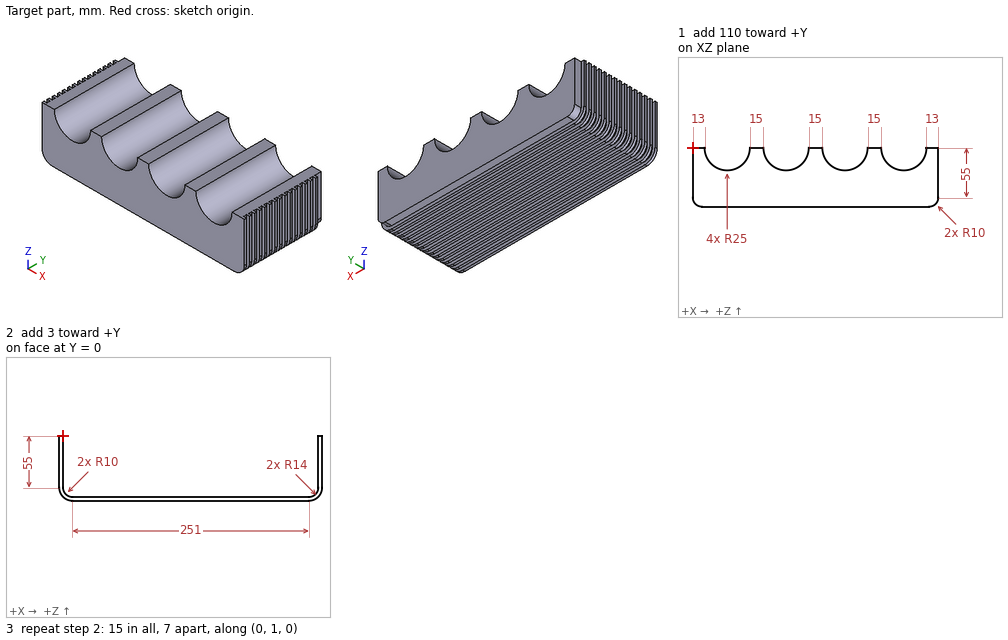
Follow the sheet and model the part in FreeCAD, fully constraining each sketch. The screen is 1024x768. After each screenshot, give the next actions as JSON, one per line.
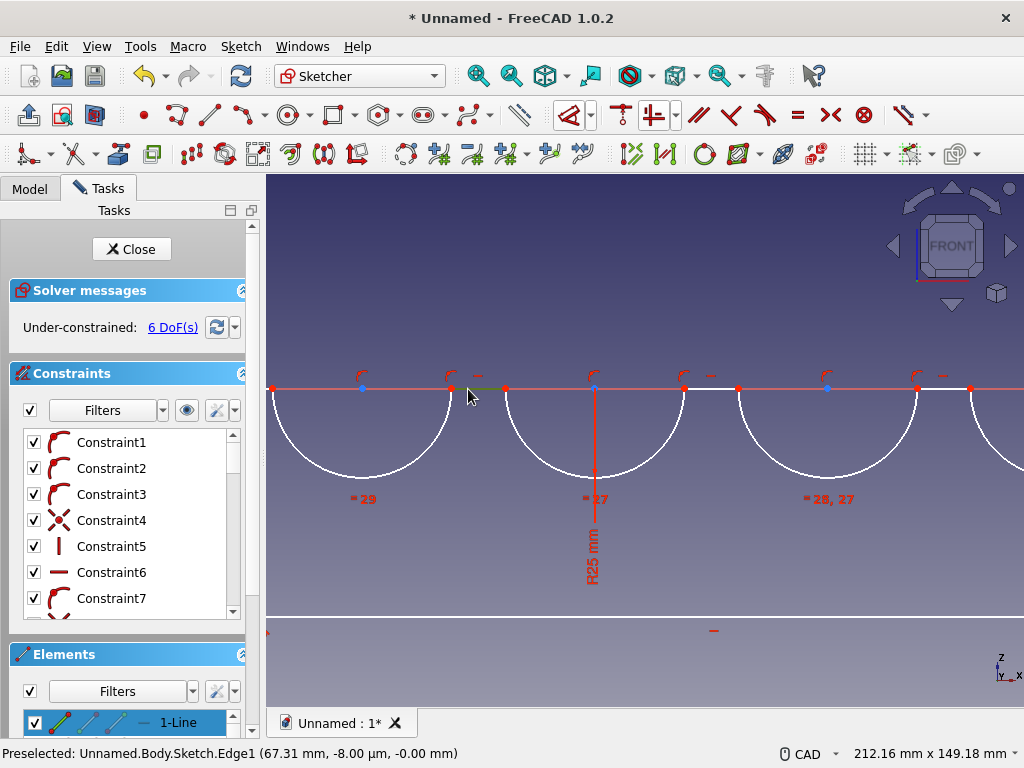
{"action": "left_click", "coordinate": [590, 116]}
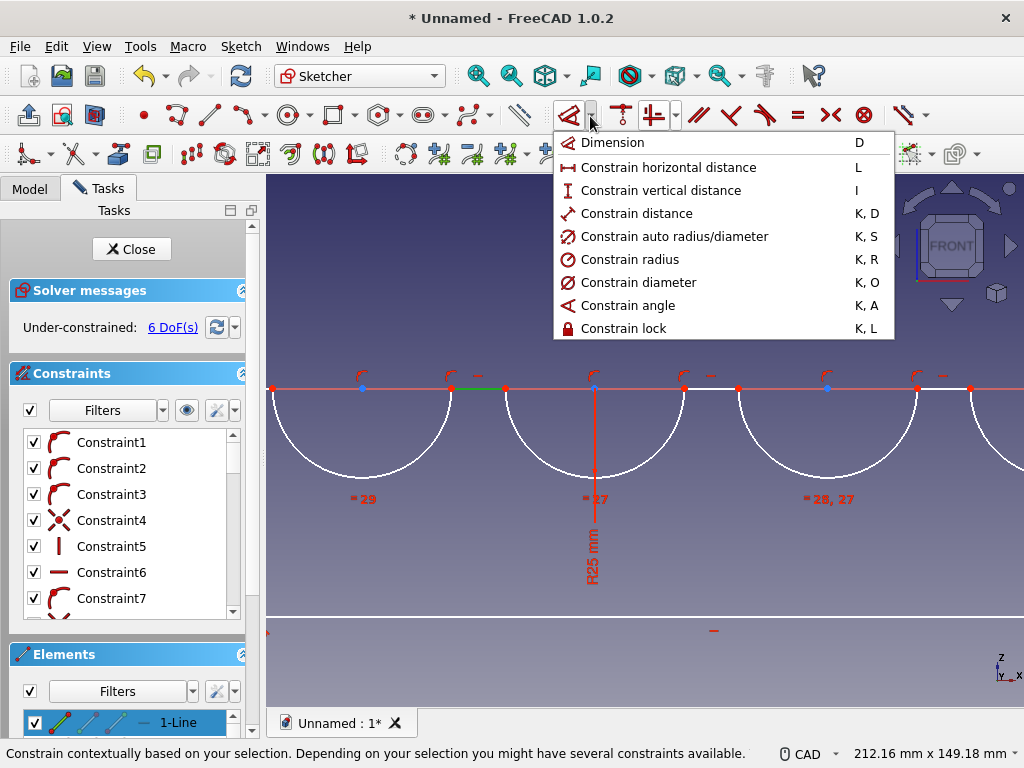
{"action": "left_click", "coordinate": [724, 168]}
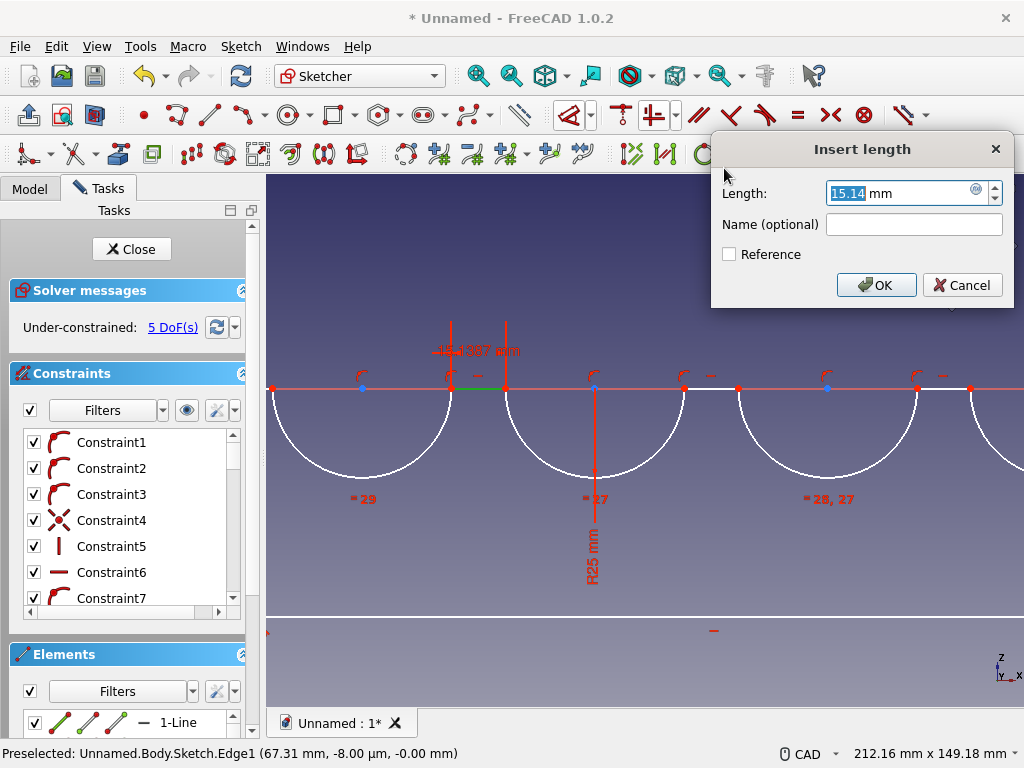
{"action": "type", "text": "15"}
{"action": "key", "text": "Return"}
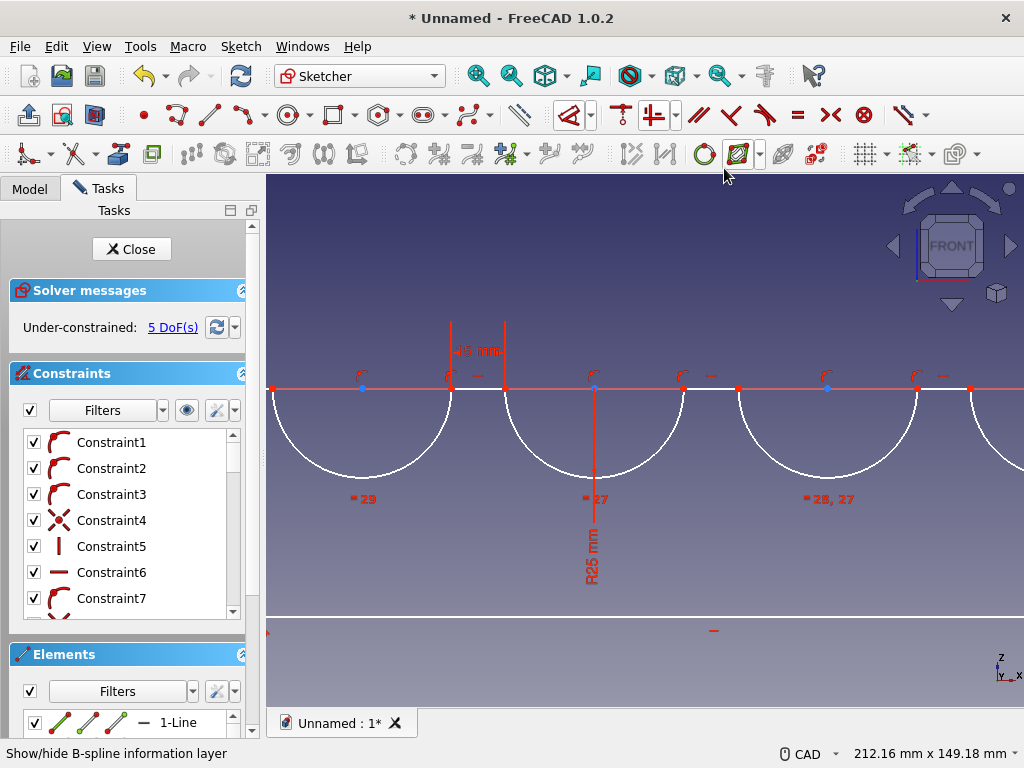
{"action": "left_click", "coordinate": [700, 389]}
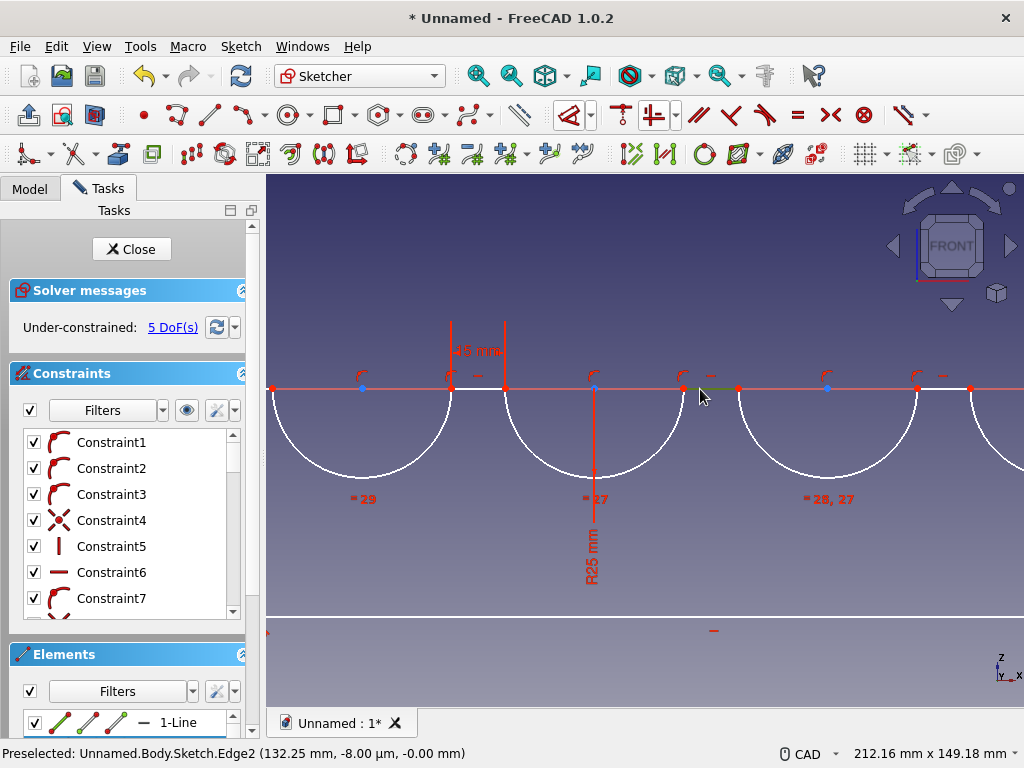
{"action": "left_click", "coordinate": [590, 116]}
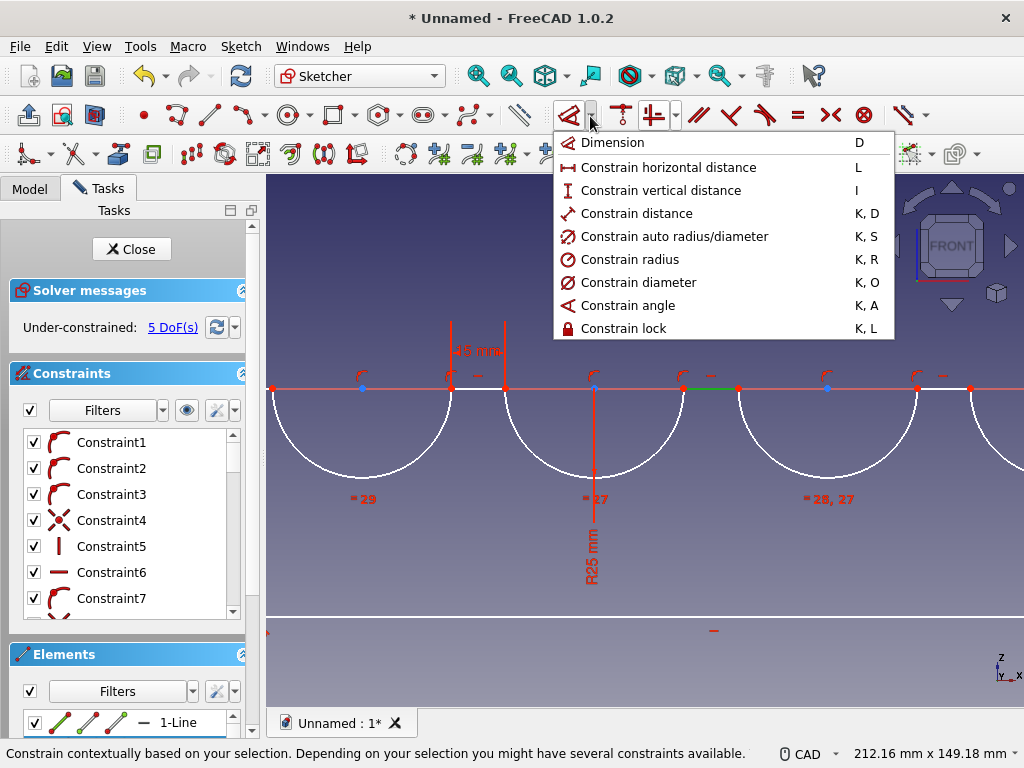
{"action": "left_click", "coordinate": [724, 168]}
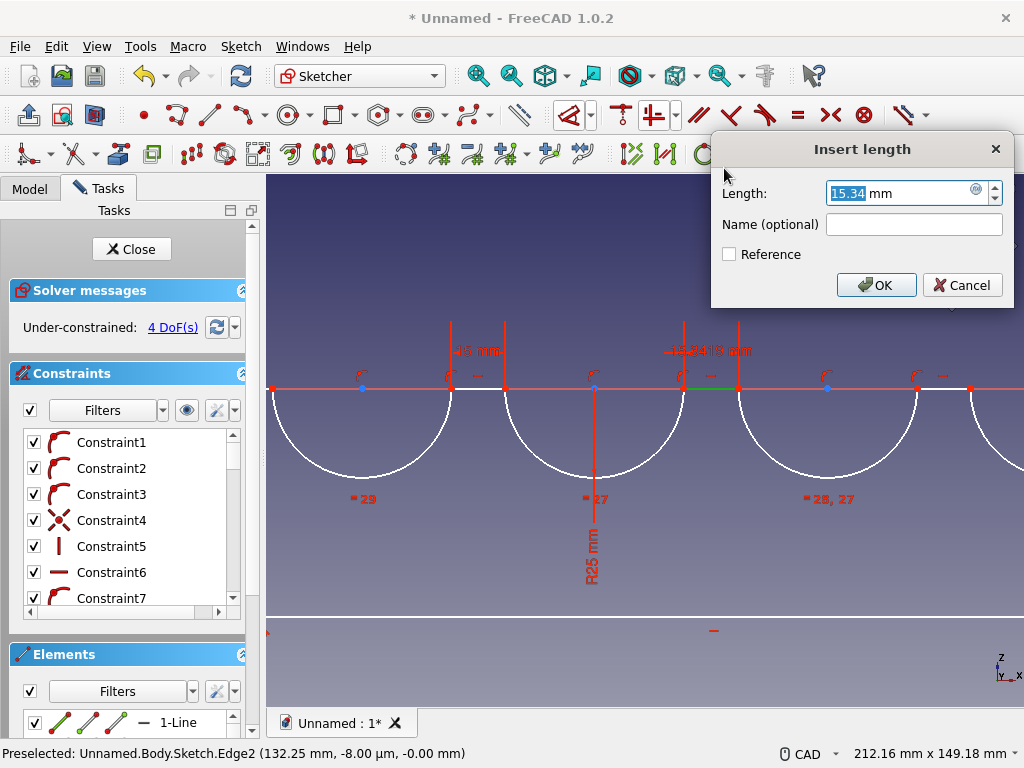
{"action": "type", "text": "15"}
{"action": "key", "text": "Return"}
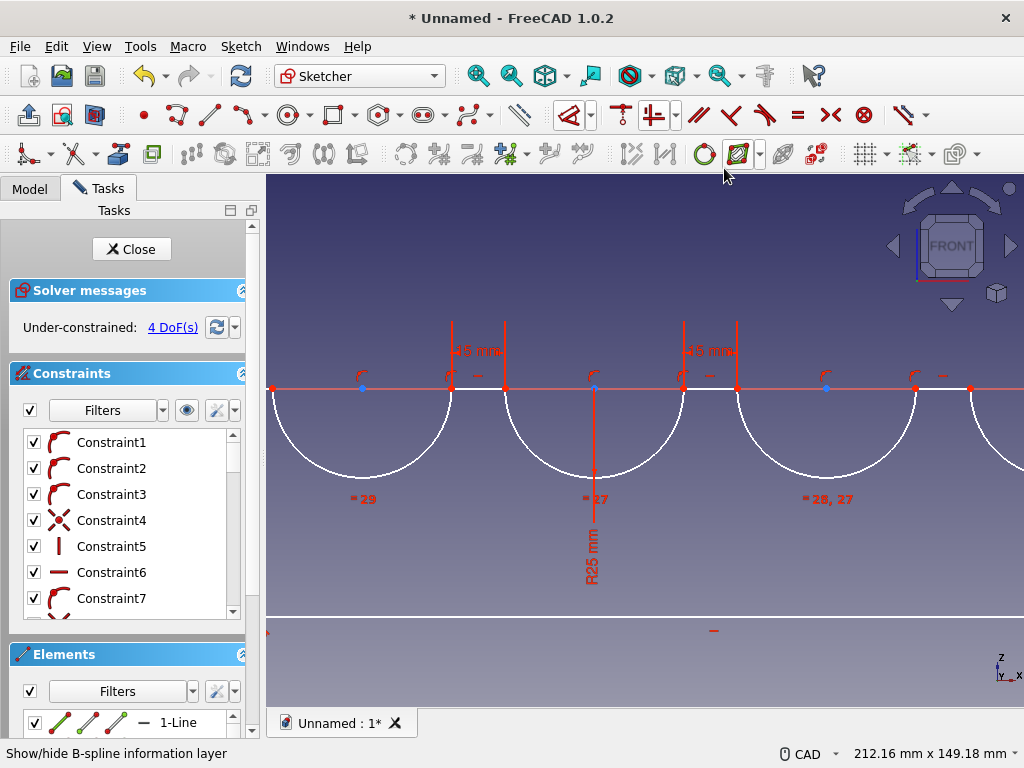
{"action": "scroll", "coordinate": [466, 388], "scroll_direction": "down", "scroll_amount": 4}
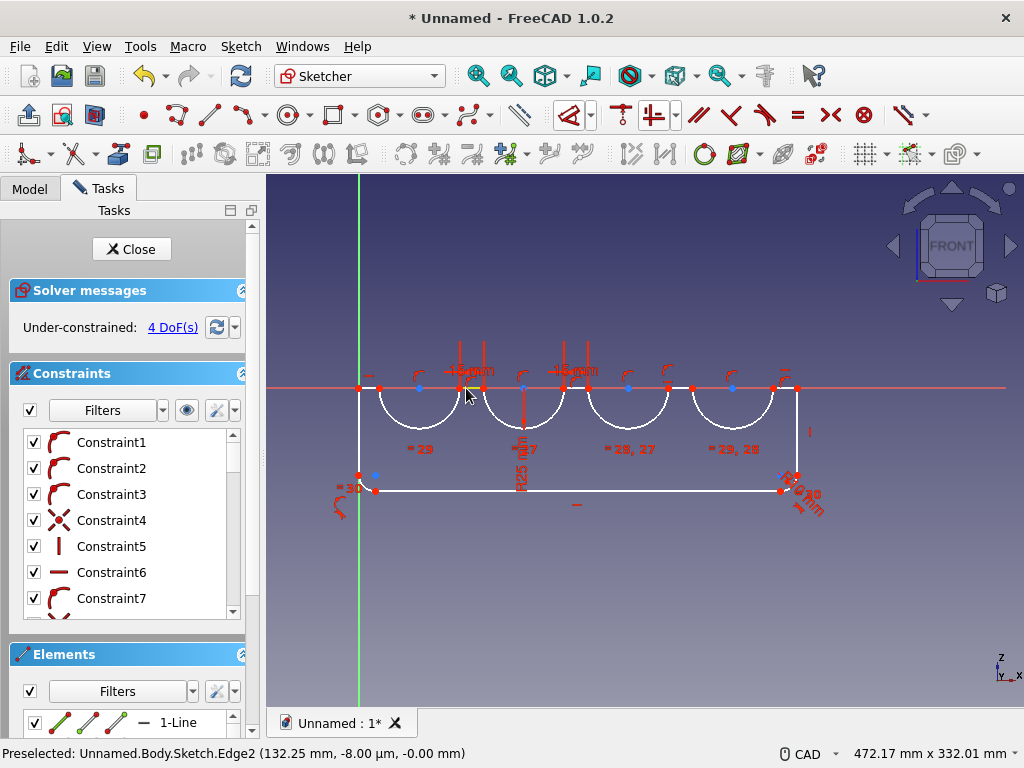
{"action": "scroll", "coordinate": [676, 388], "scroll_direction": "up", "scroll_amount": 4}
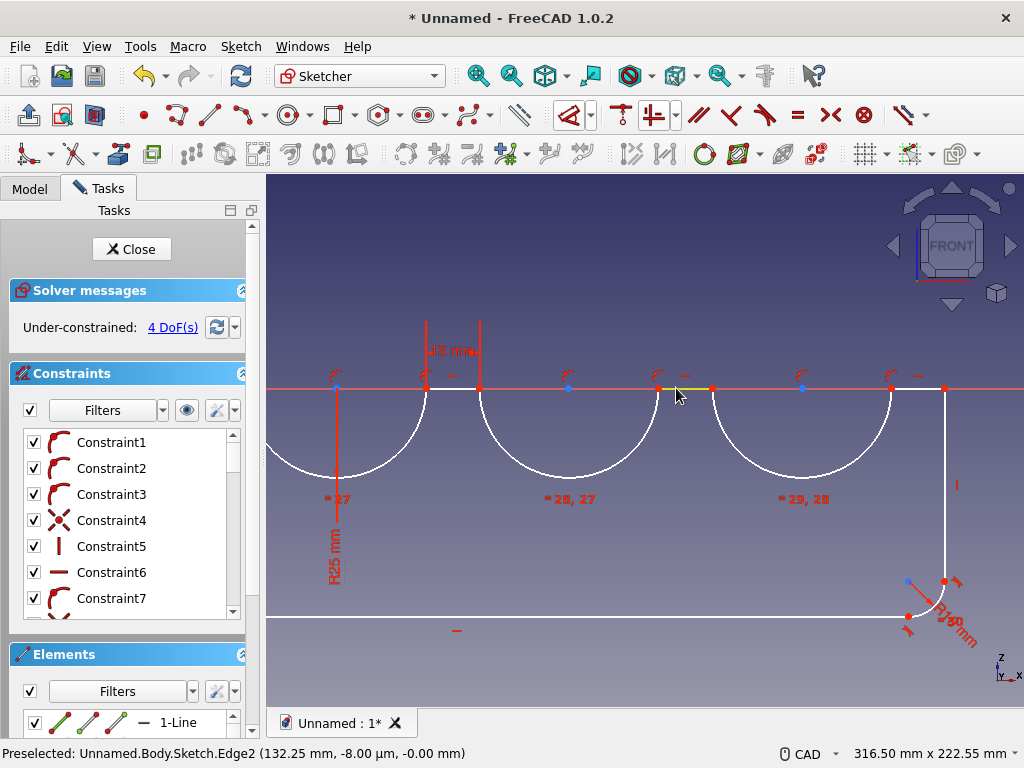
{"action": "left_click", "coordinate": [675, 389]}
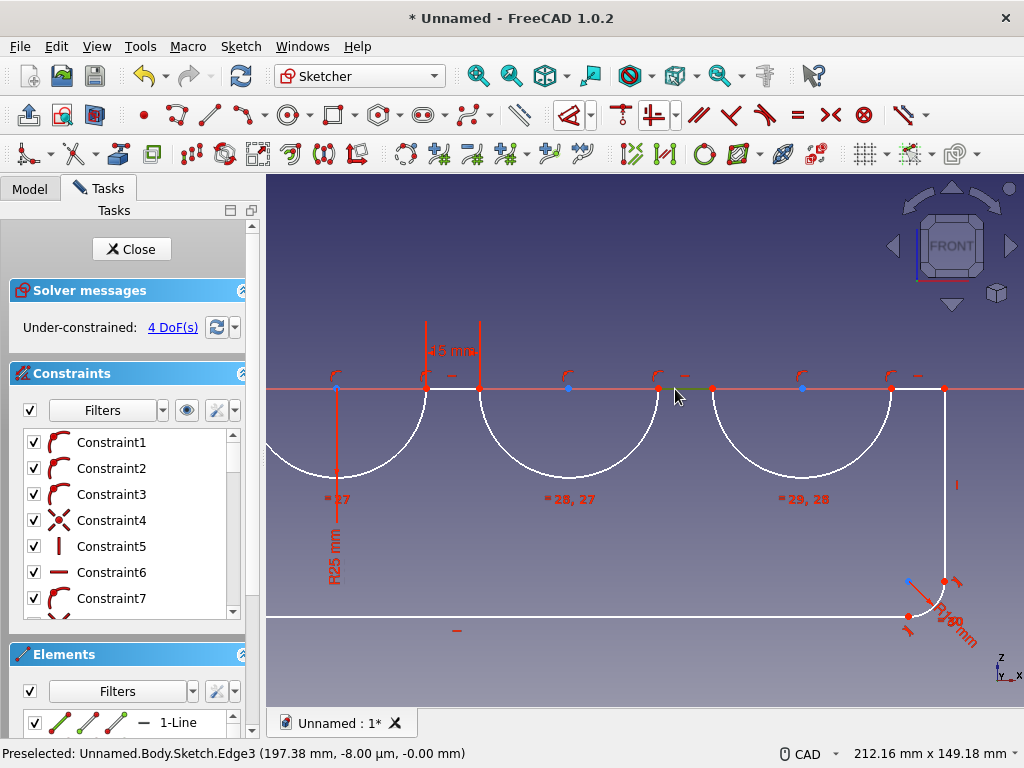
{"action": "key", "text": "l"}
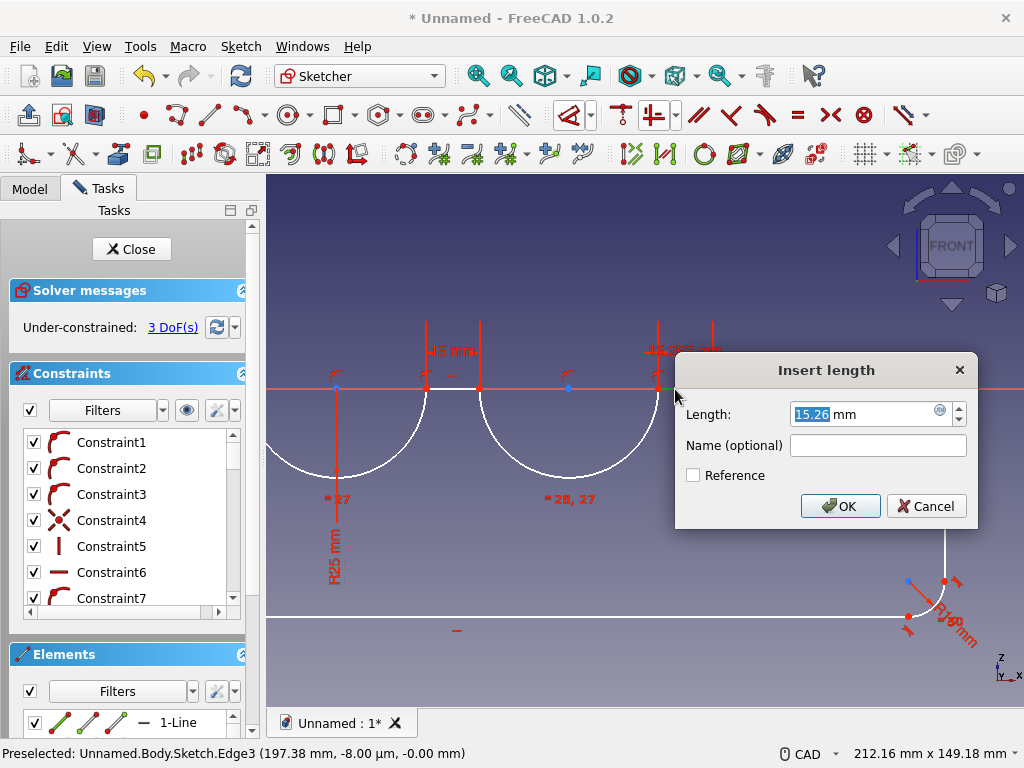
{"action": "type", "text": "15"}
{"action": "key", "text": "Return"}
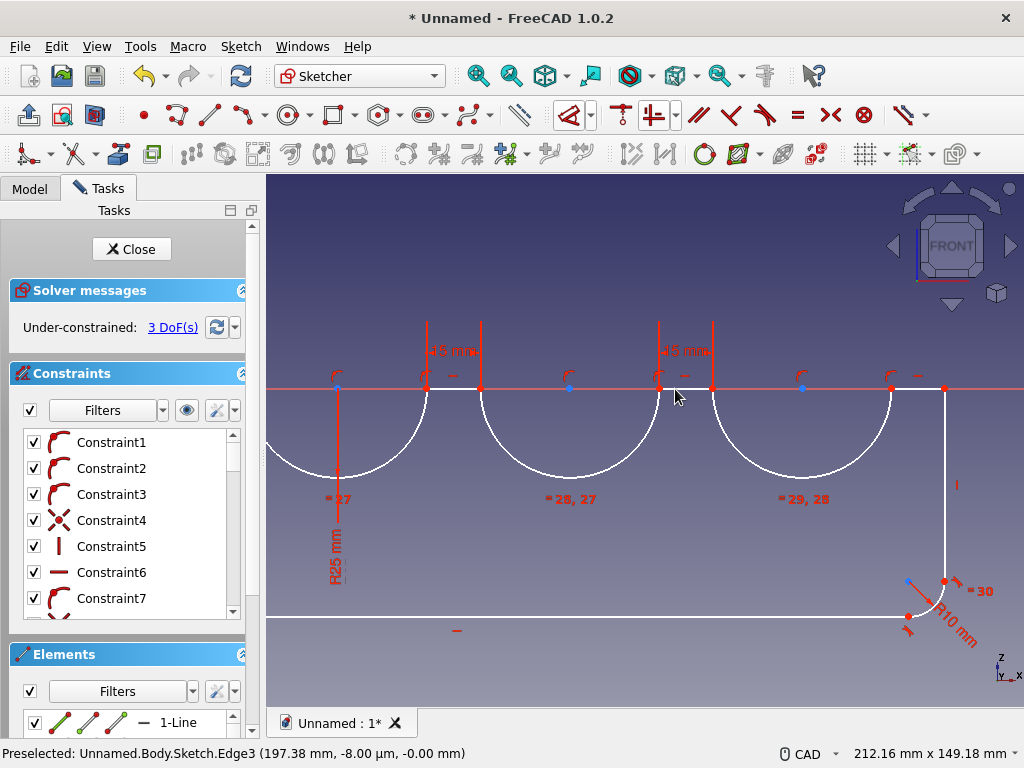
{"action": "scroll", "coordinate": [677, 388], "scroll_direction": "down", "scroll_amount": 4}